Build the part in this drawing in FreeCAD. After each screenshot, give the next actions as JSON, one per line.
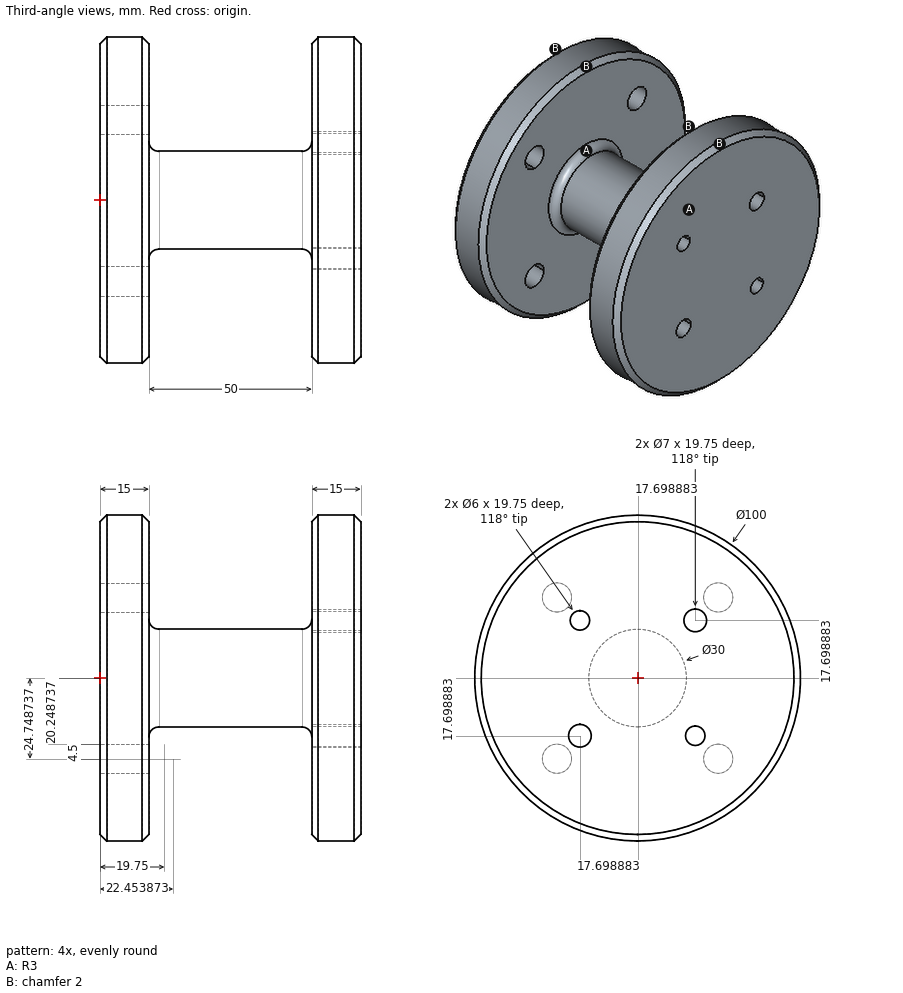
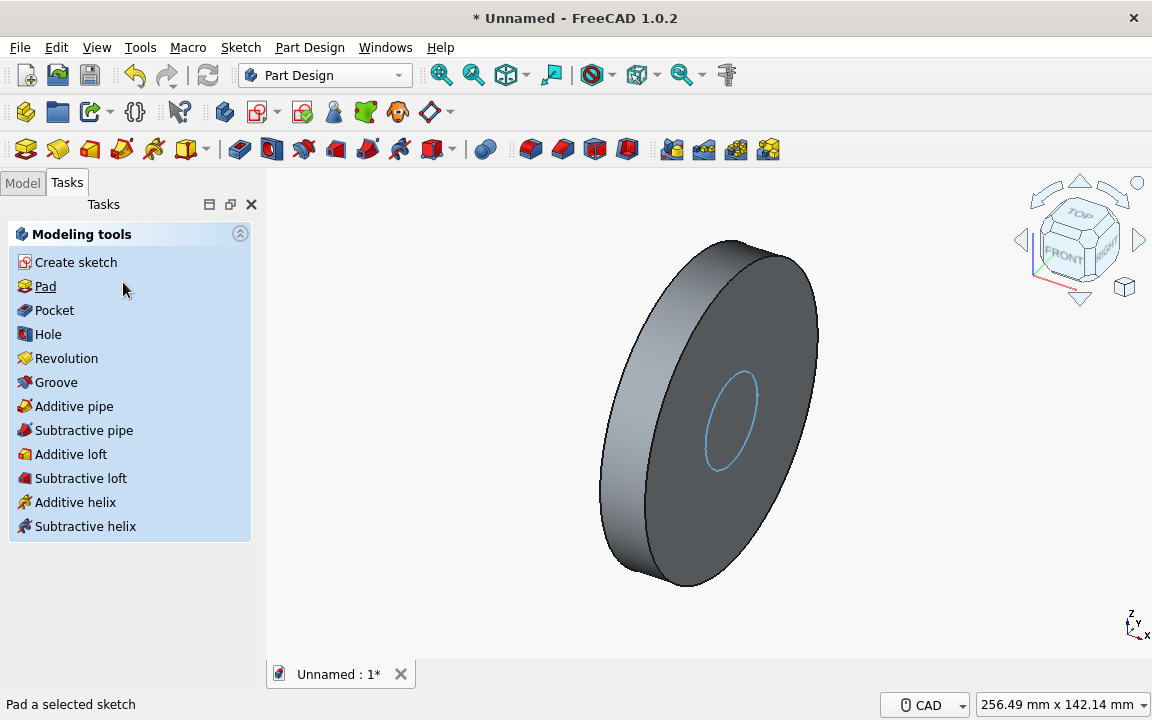
{"action": "left_click", "coordinate": [26, 150]}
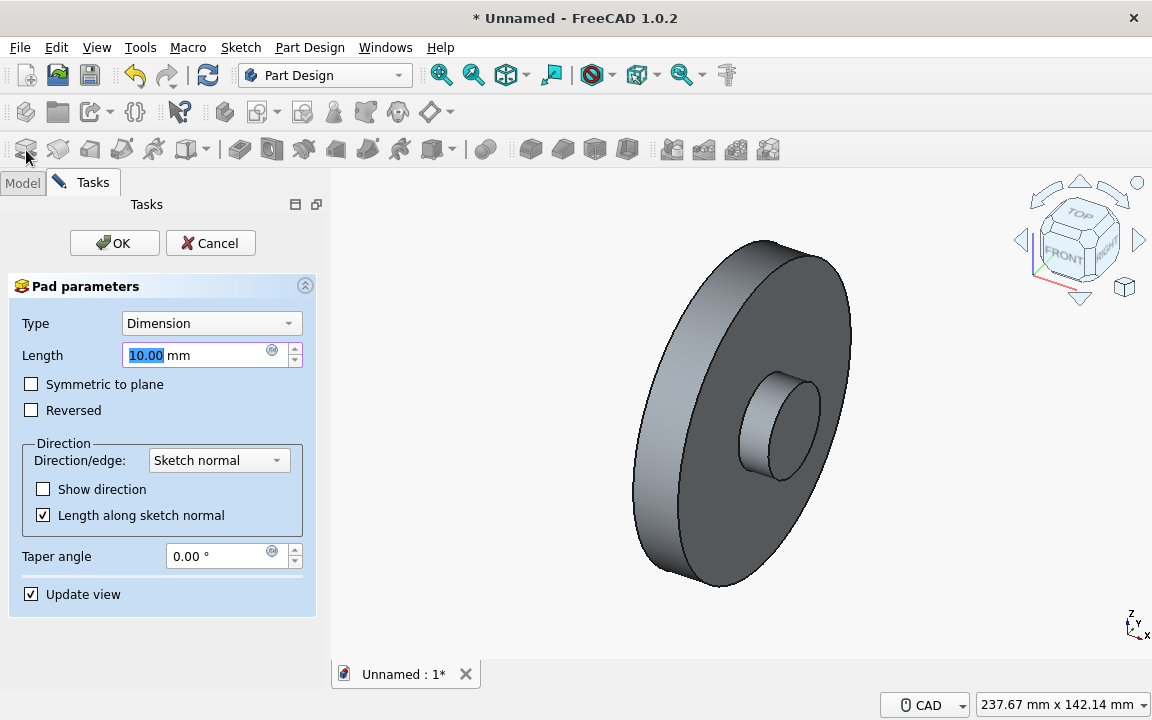
{"action": "type", "text": "50"}
{"action": "key", "text": "Tab"}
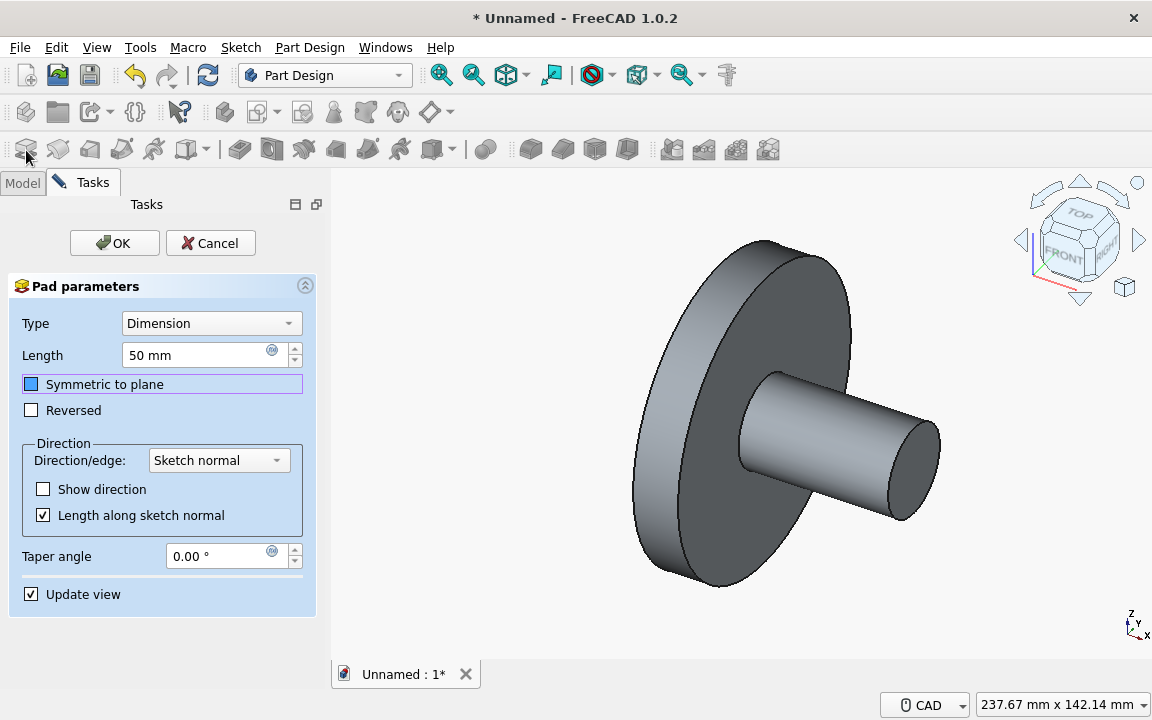
{"action": "left_click", "coordinate": [115, 243]}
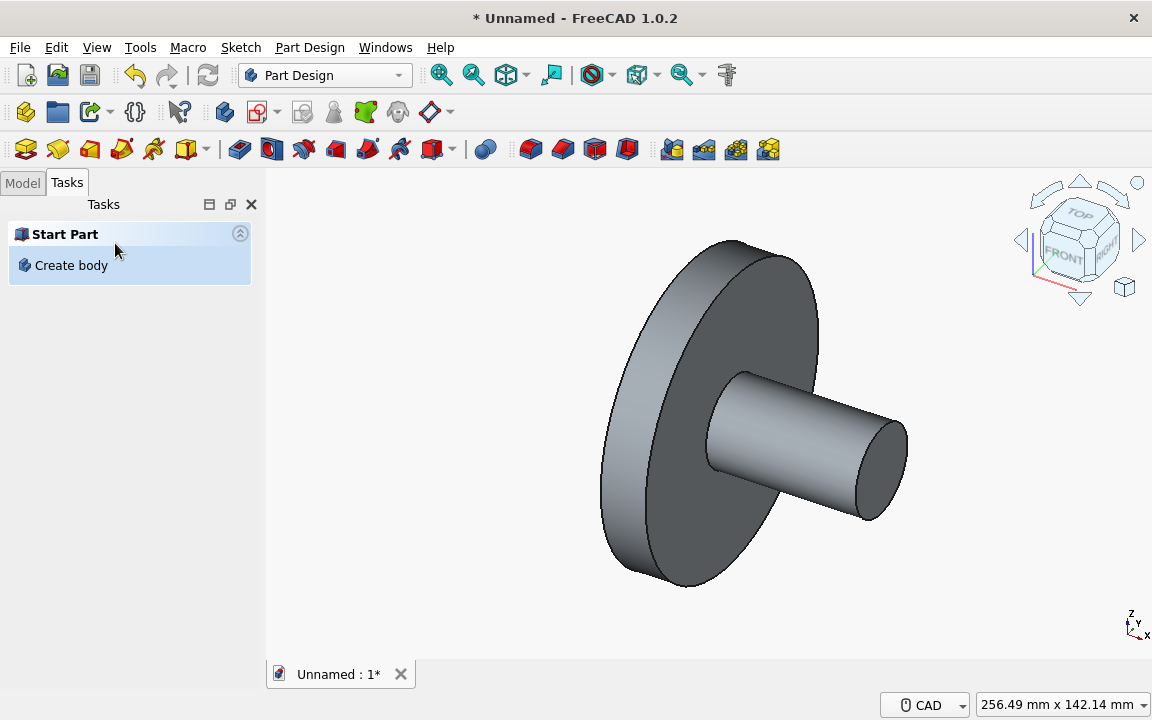
{"action": "left_click", "coordinate": [442, 76]}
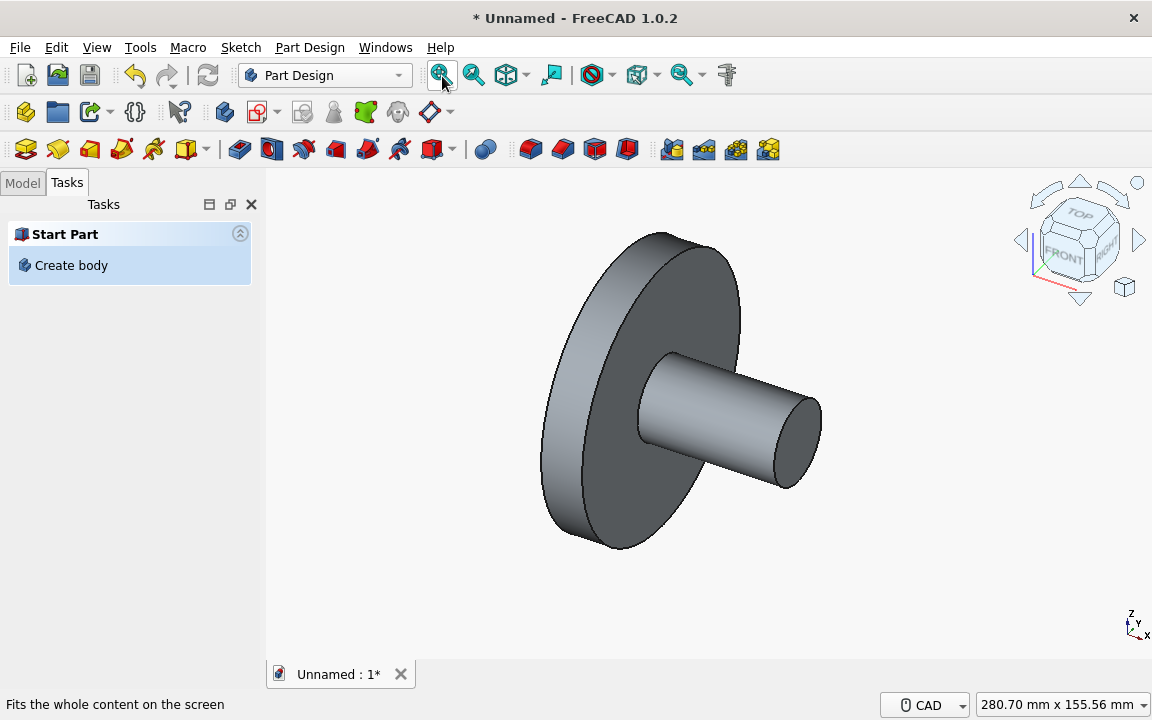
{"action": "left_click", "coordinate": [798, 442]}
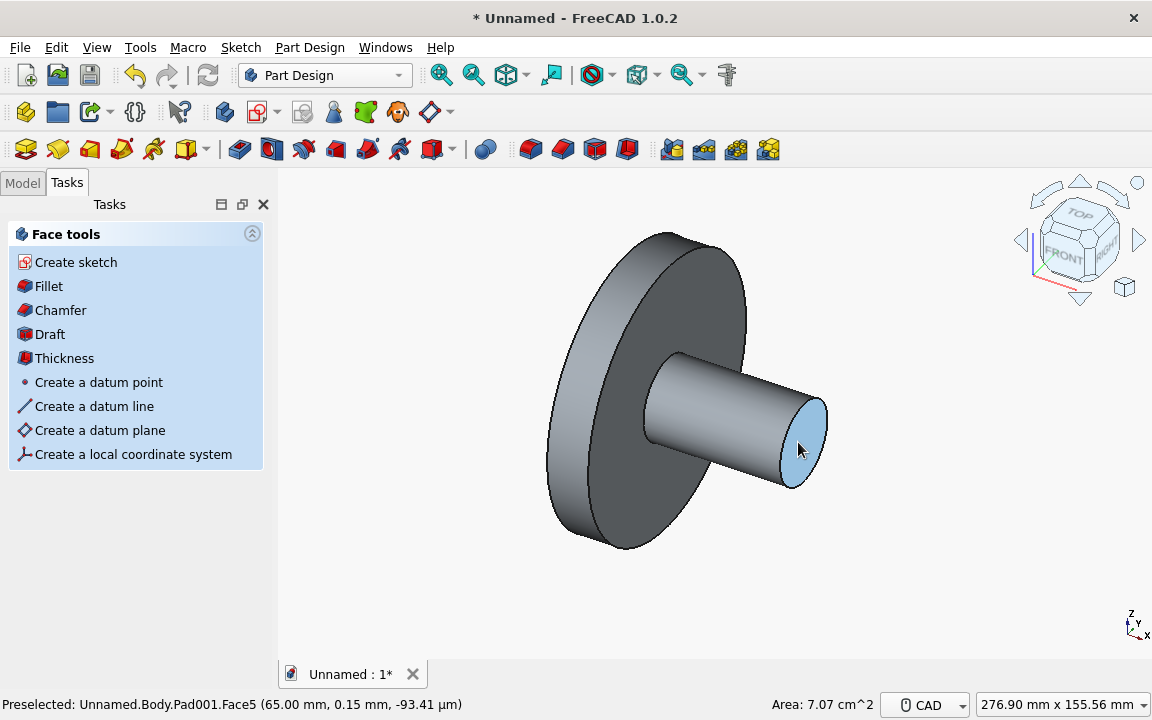
{"action": "left_click", "coordinate": [258, 112]}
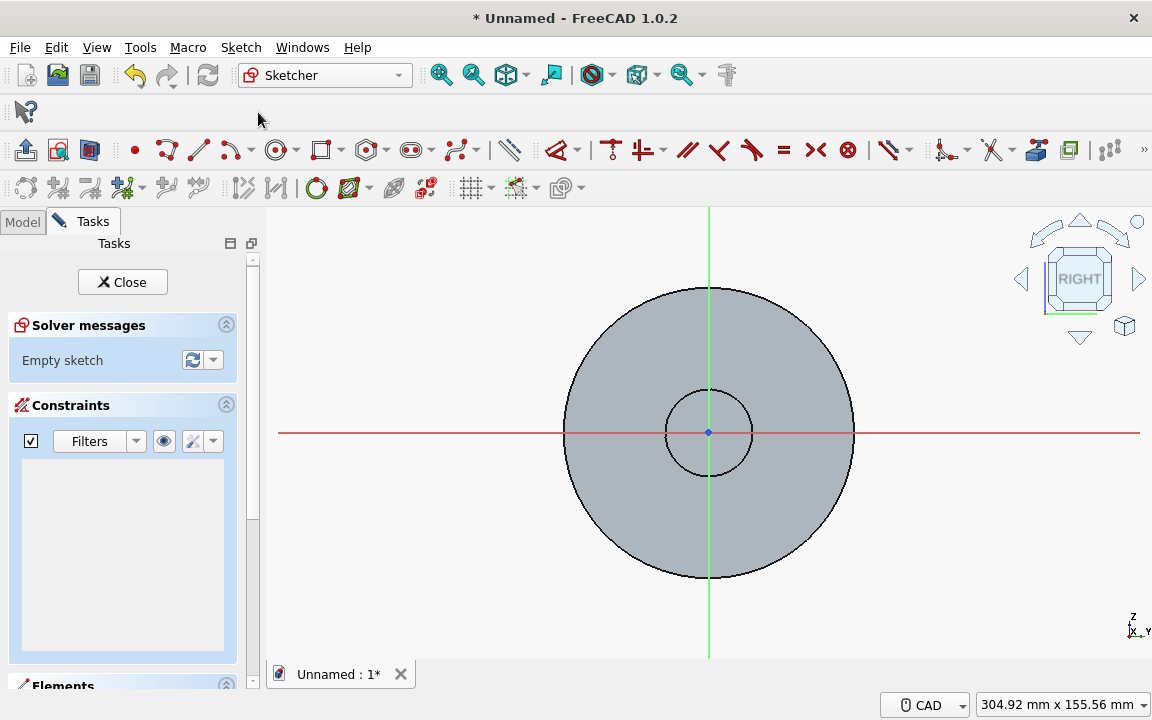
{"action": "key", "text": "g c"}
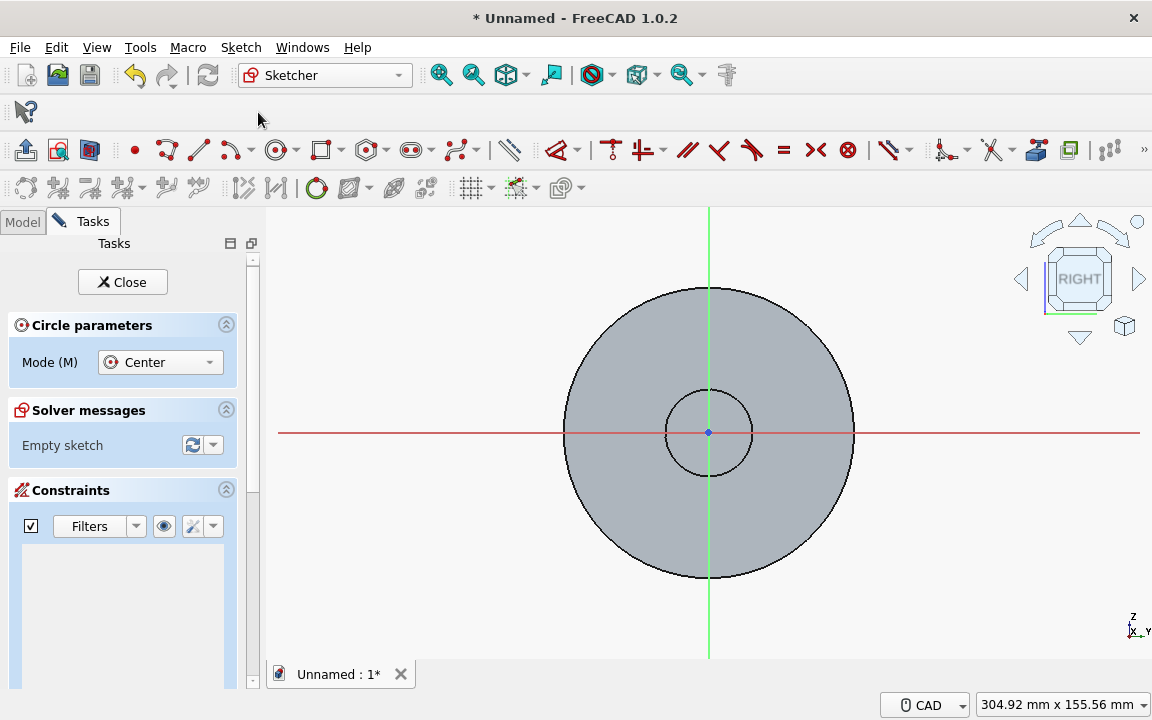
{"action": "left_click", "coordinate": [709, 433]}
{"action": "left_click", "coordinate": [812, 330]}
{"action": "key", "text": "Escape"}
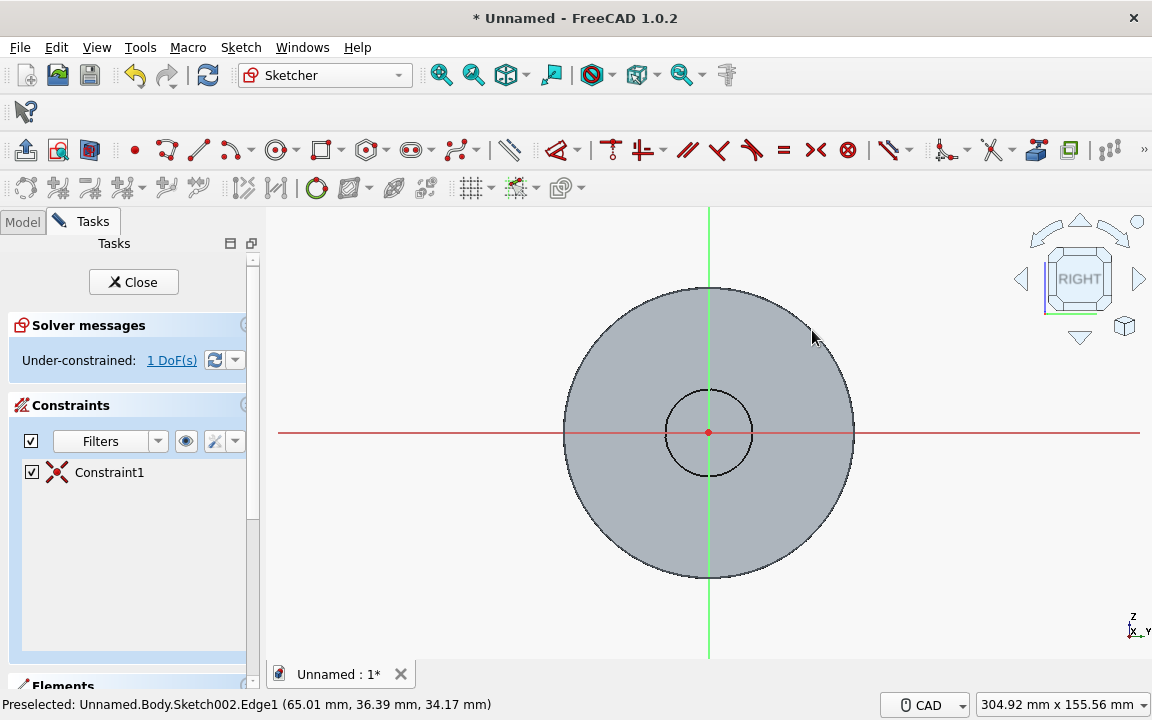
{"action": "left_click", "coordinate": [556, 150]}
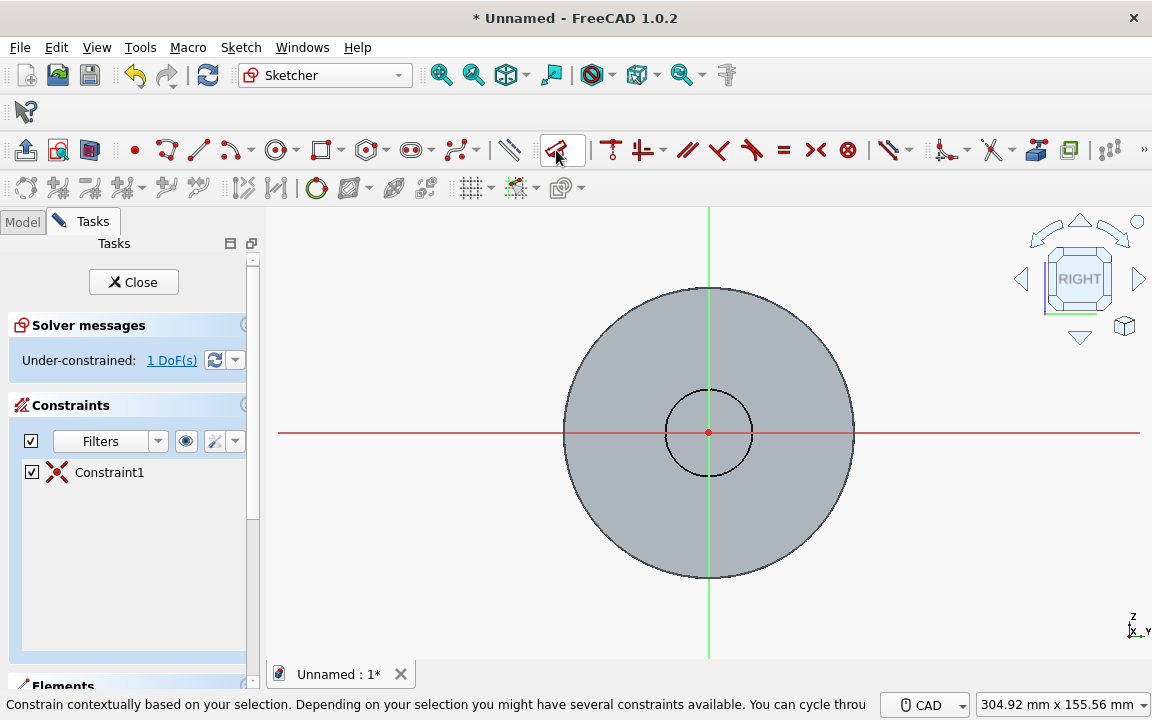
{"action": "left_click", "coordinate": [811, 330]}
{"action": "left_click", "coordinate": [834, 307]}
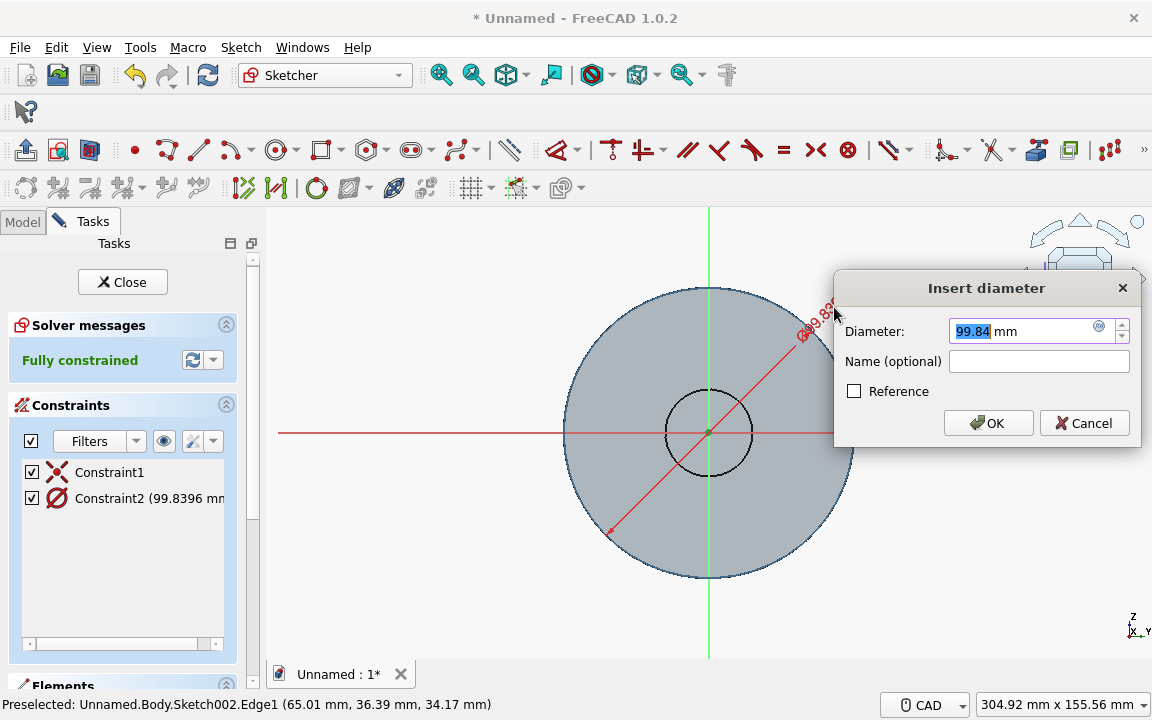
{"action": "type", "text": "100"}
{"action": "key", "text": "Return"}
{"action": "key", "text": "Escape"}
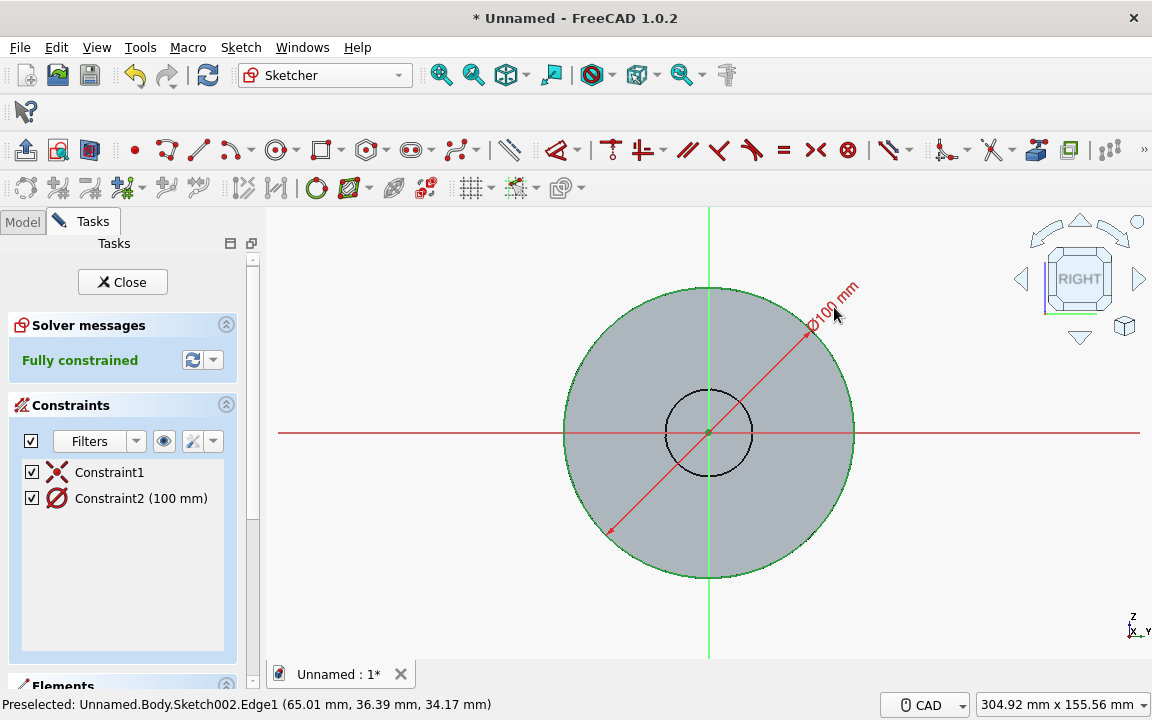
{"action": "left_click", "coordinate": [123, 282]}